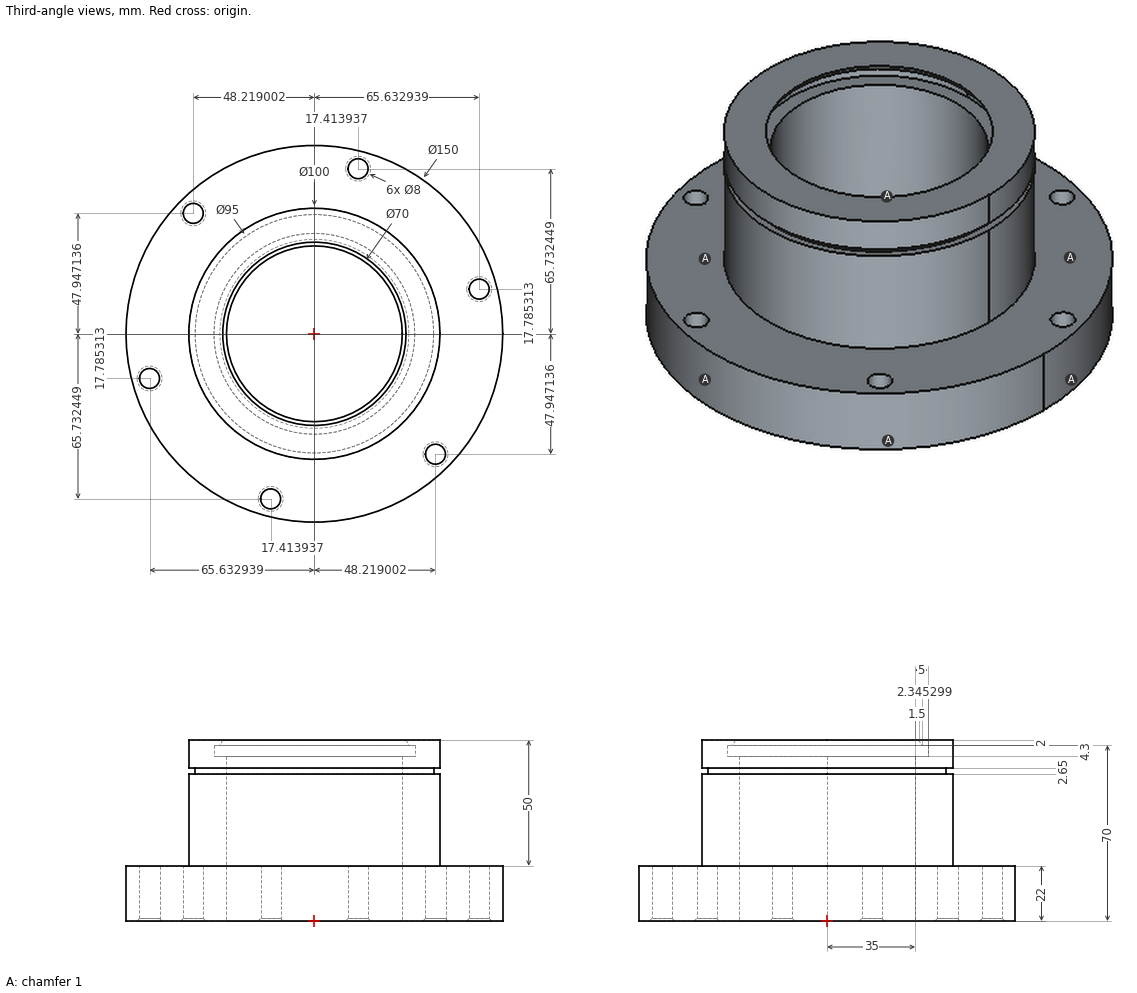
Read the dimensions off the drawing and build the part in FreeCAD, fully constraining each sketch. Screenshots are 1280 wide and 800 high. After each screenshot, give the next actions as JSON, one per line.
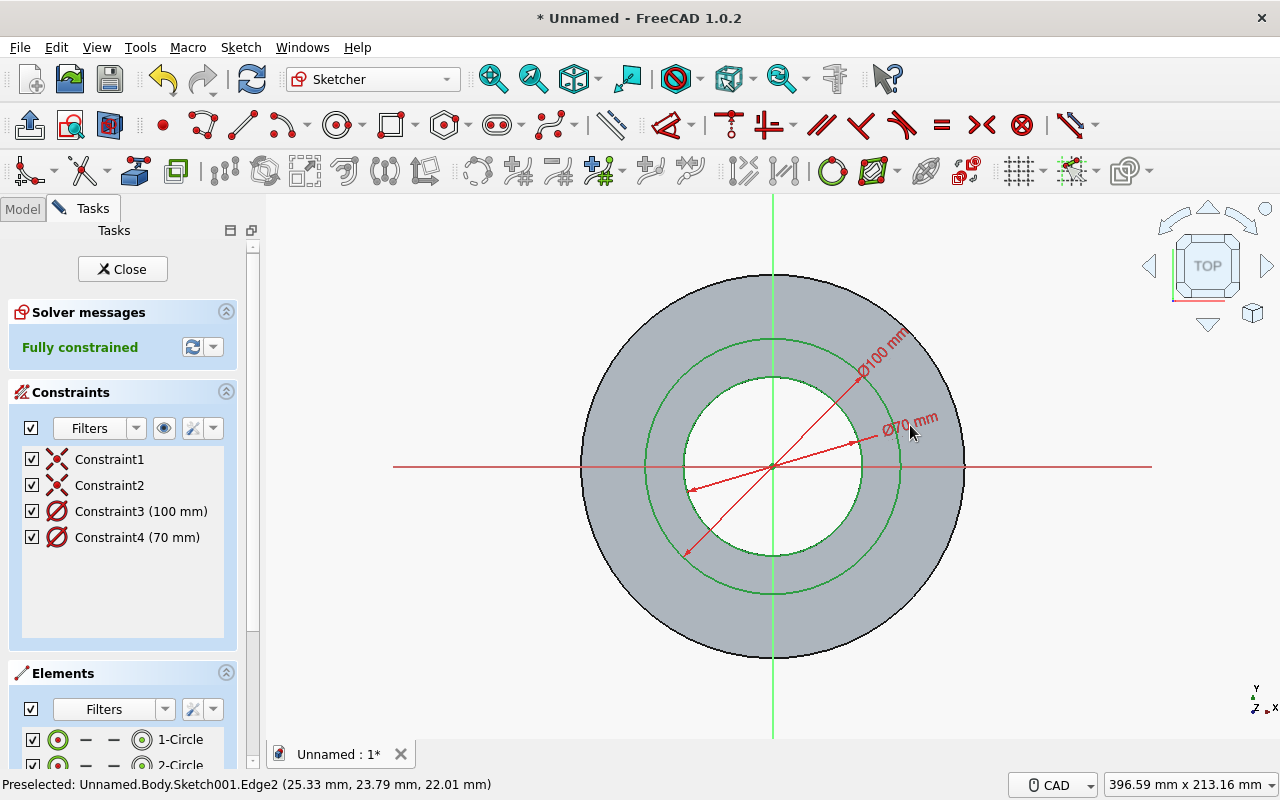
{"action": "left_click", "coordinate": [123, 269]}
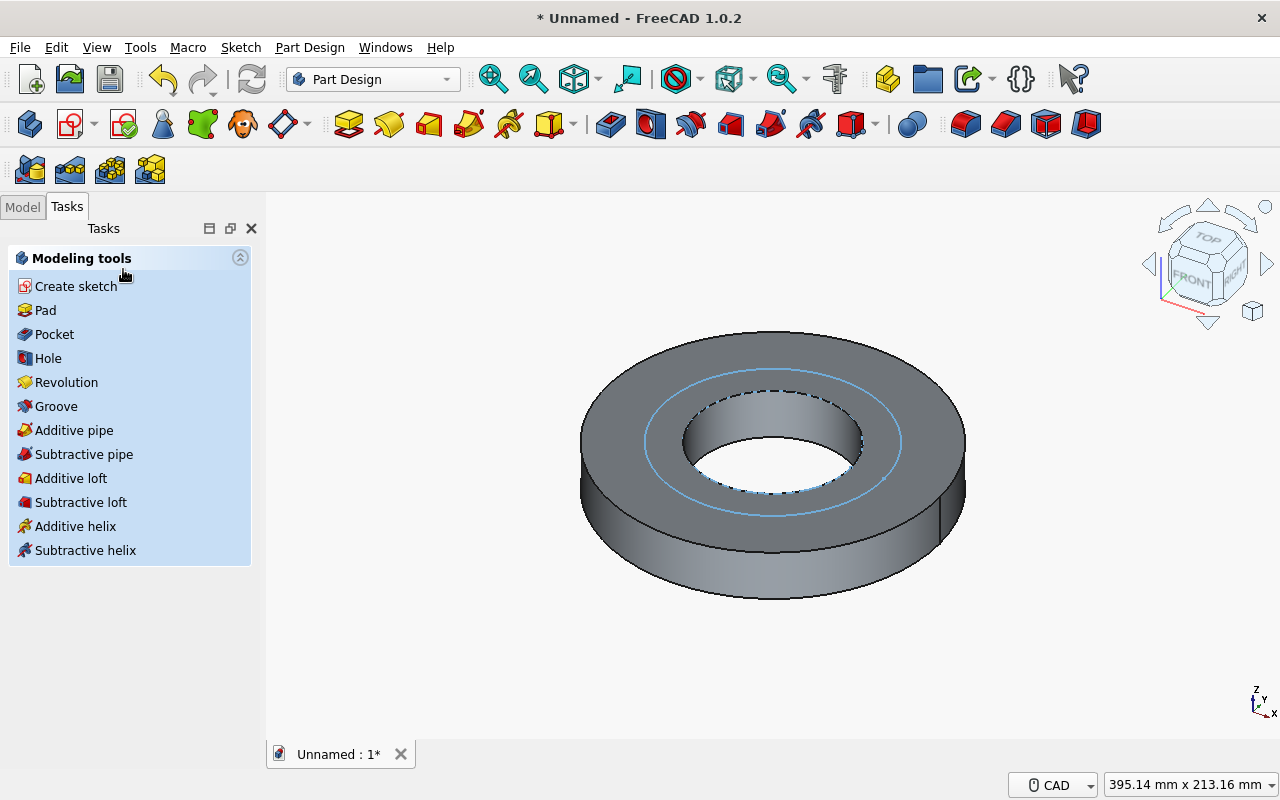
{"action": "left_click", "coordinate": [350, 124]}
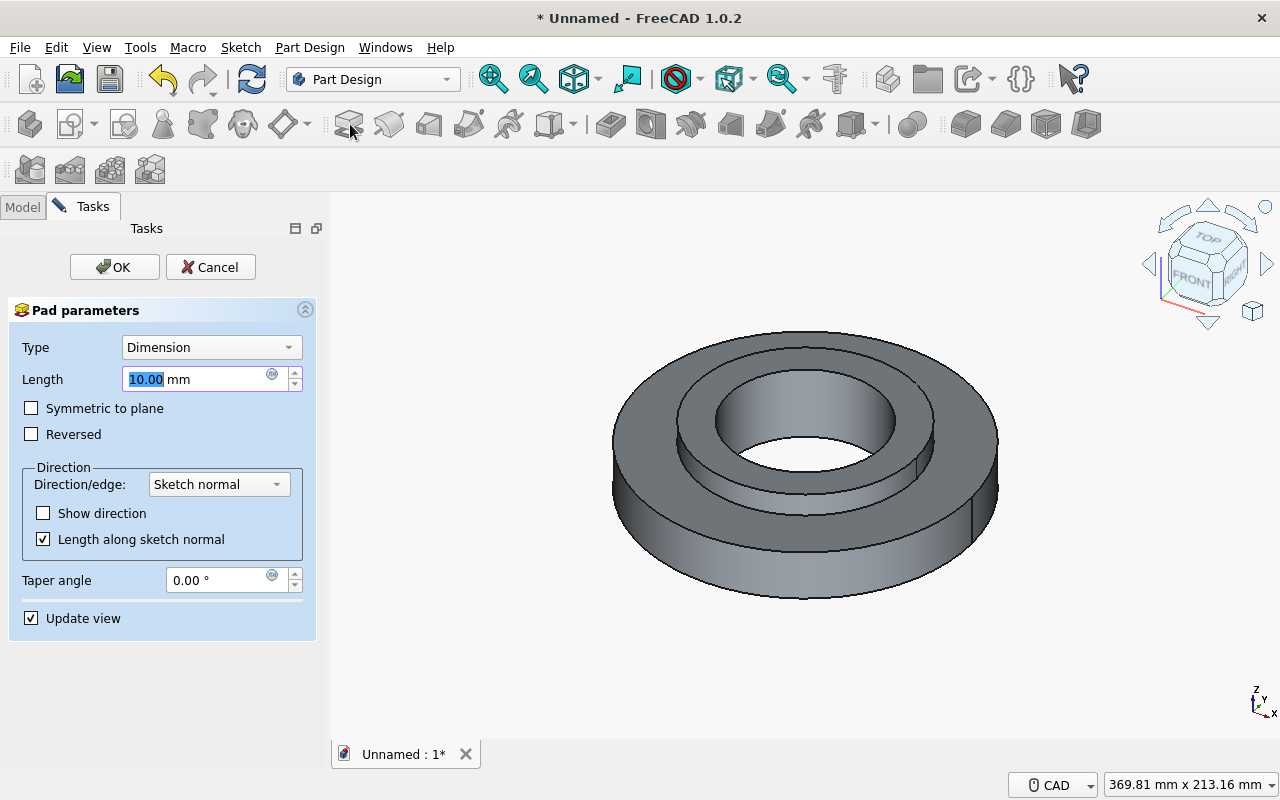
{"action": "type", "text": "50"}
{"action": "key", "text": "Tab"}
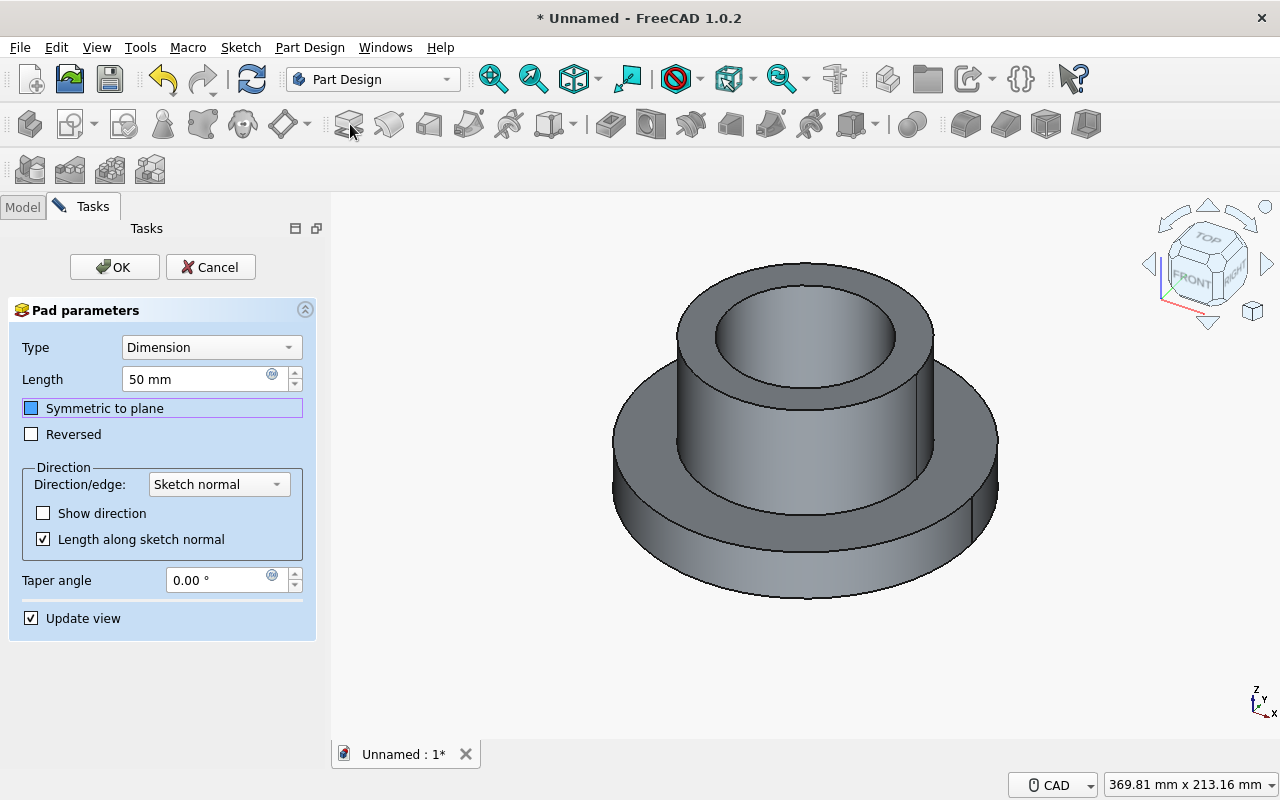
{"action": "left_click", "coordinate": [115, 267]}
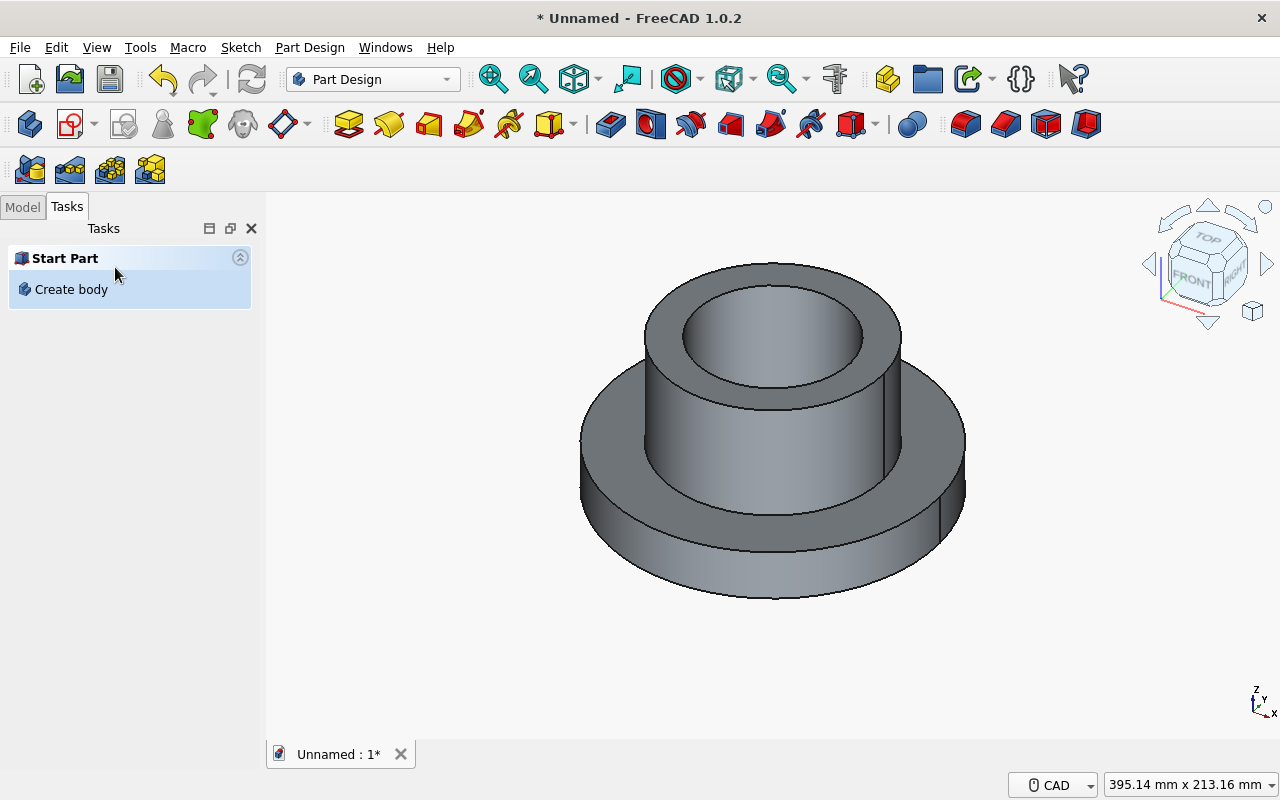
{"action": "left_click", "coordinate": [494, 80]}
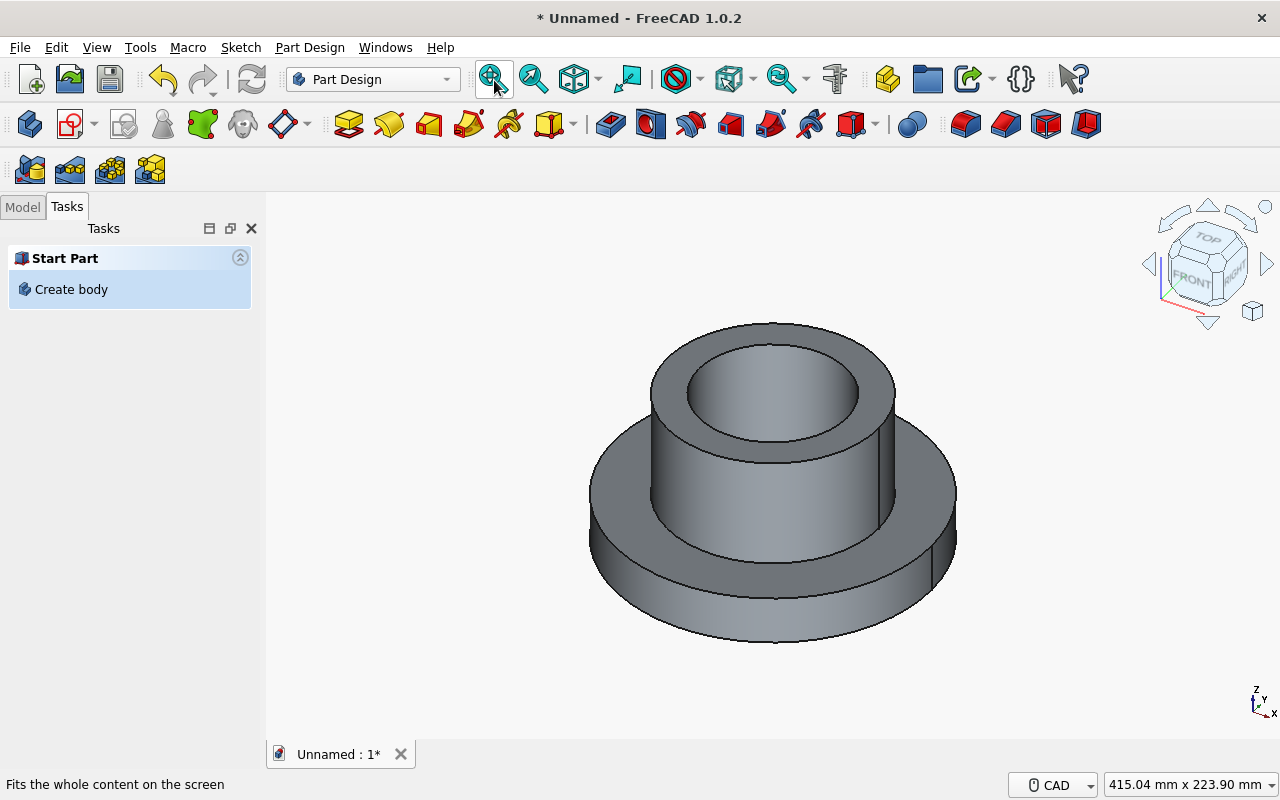
{"action": "left_click", "coordinate": [23, 206]}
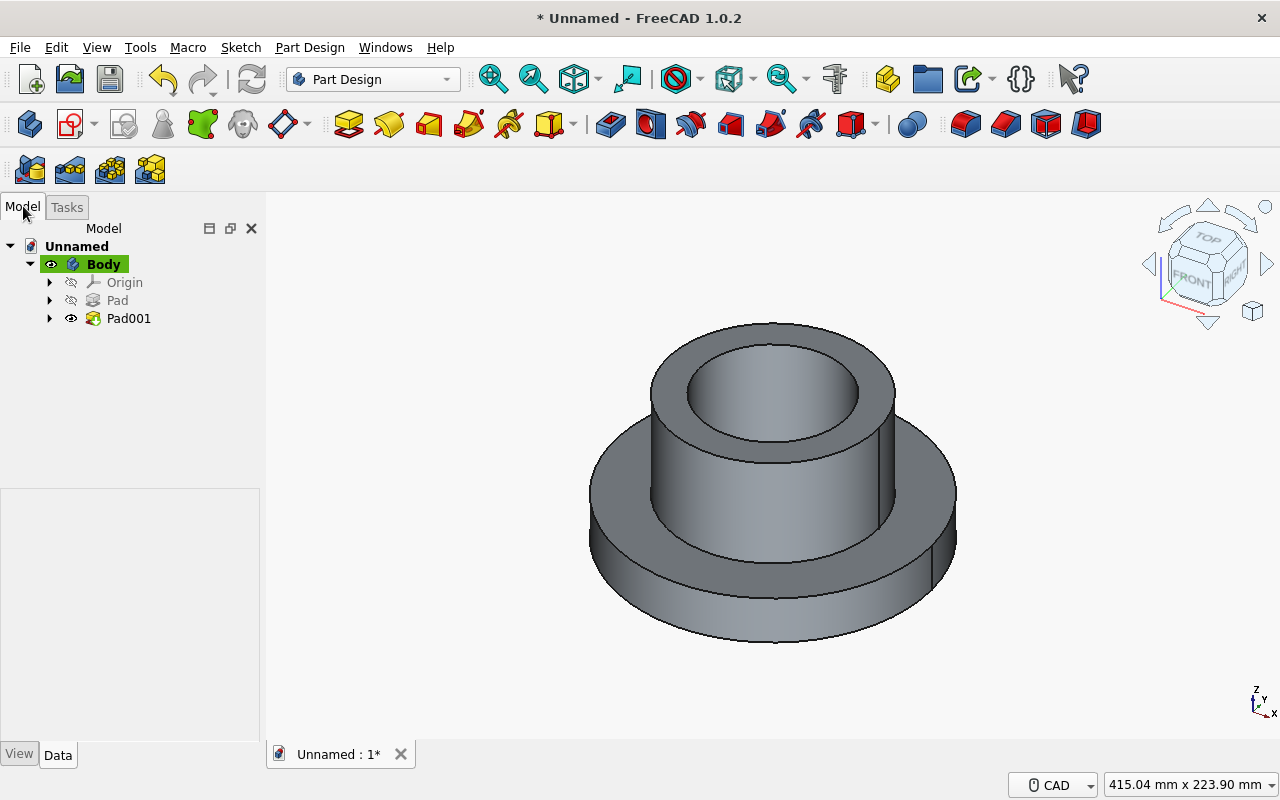
{"action": "left_click", "coordinate": [50, 282]}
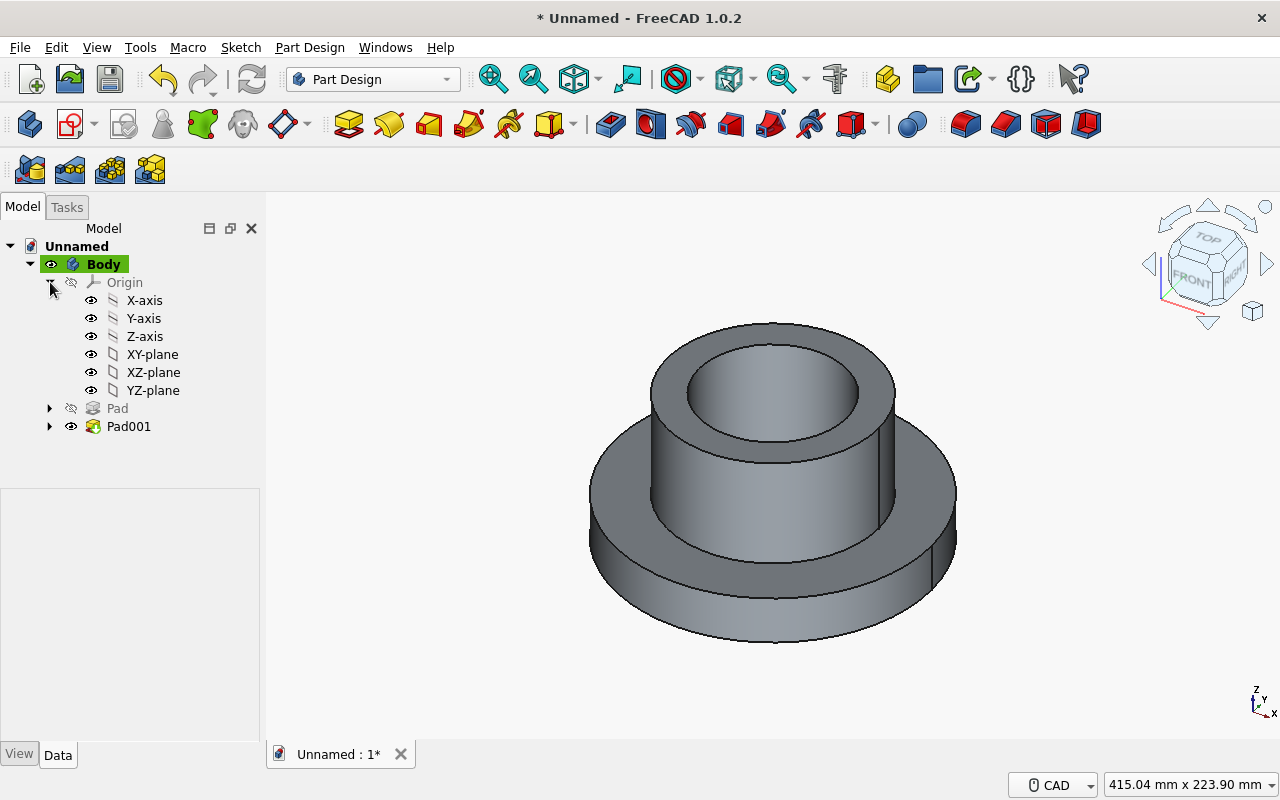
{"action": "left_click", "coordinate": [136, 354]}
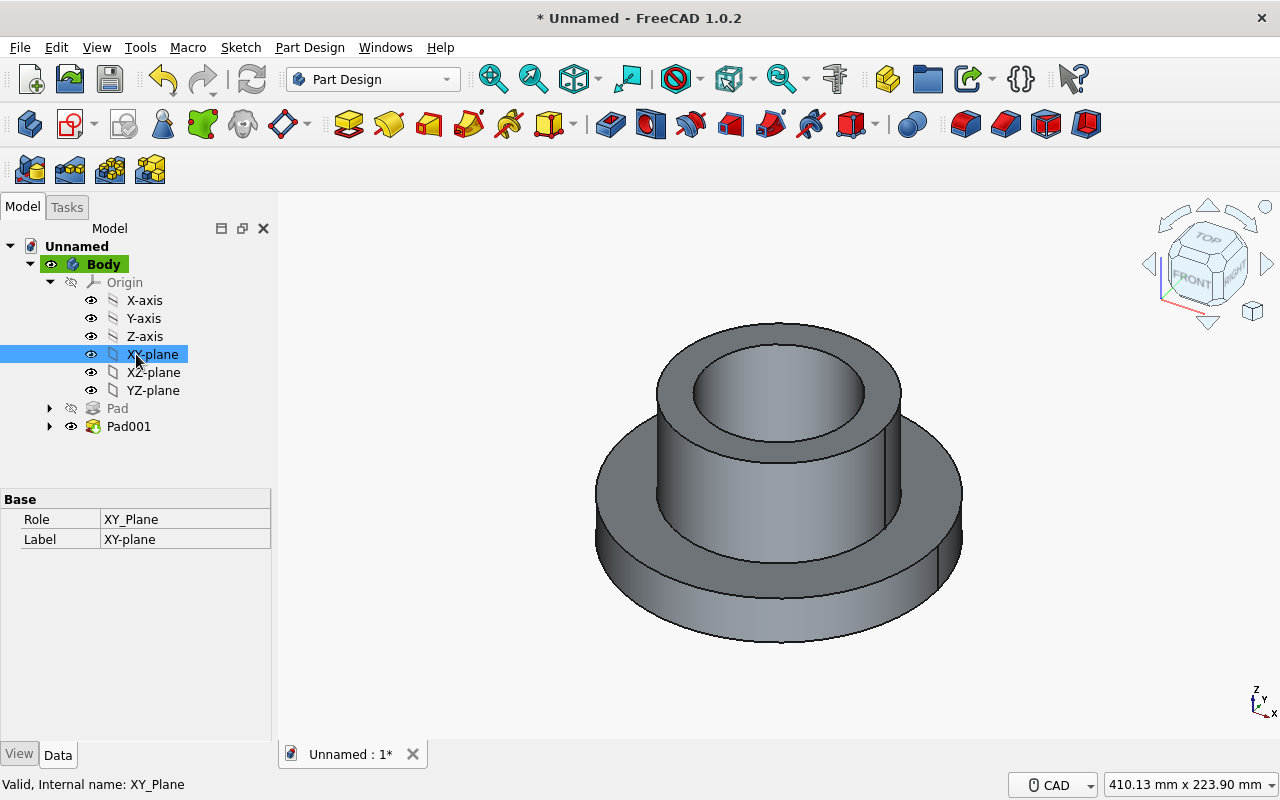
{"action": "left_click", "coordinate": [284, 124]}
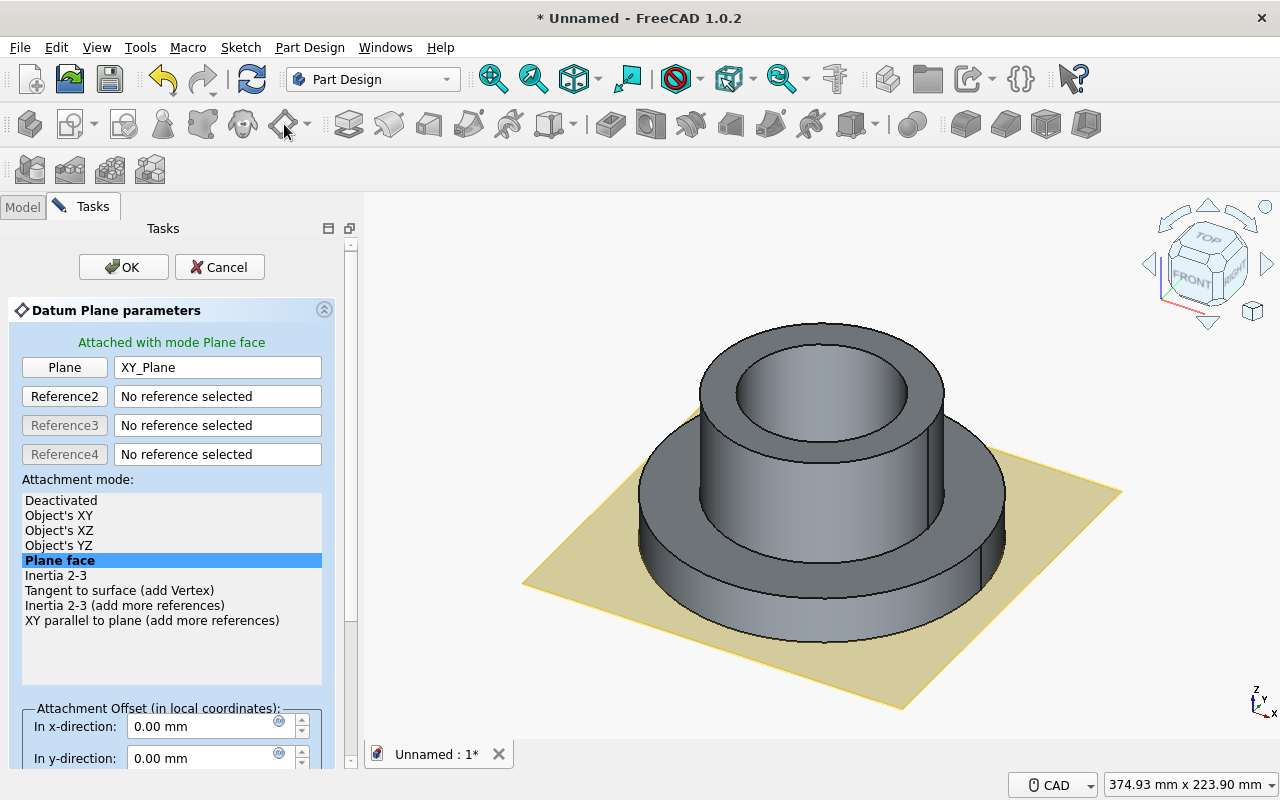
{"action": "scroll", "coordinate": [351, 503], "scroll_direction": "down", "scroll_amount": 2}